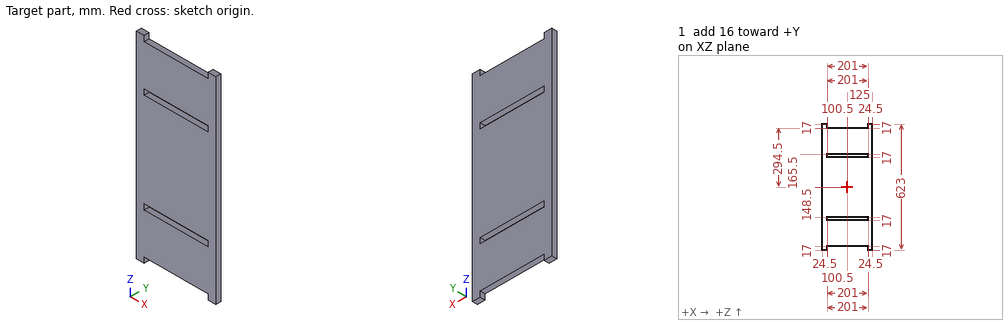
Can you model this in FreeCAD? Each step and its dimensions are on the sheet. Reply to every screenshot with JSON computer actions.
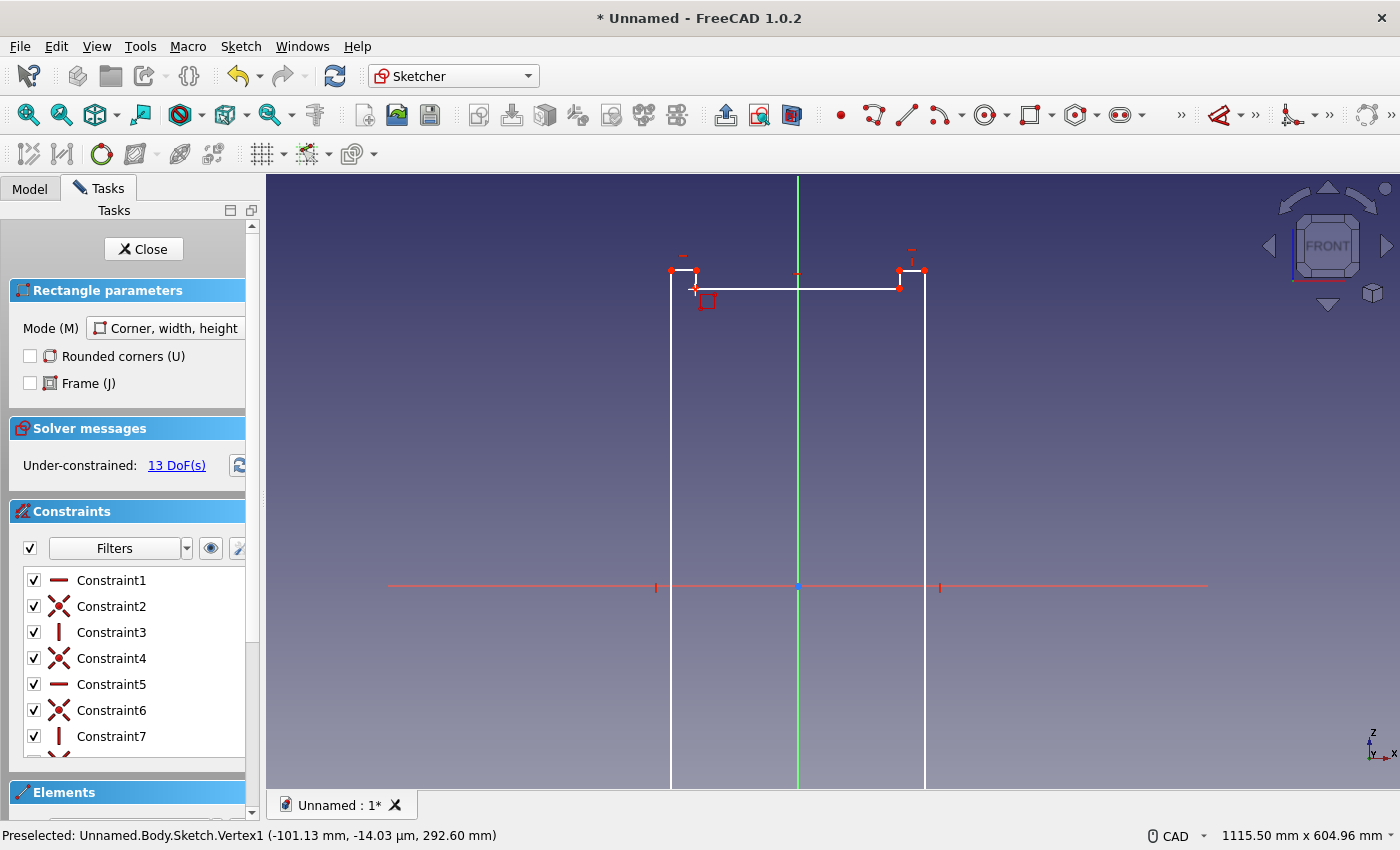
{"action": "left_click", "coordinate": [696, 418]}
{"action": "mouse_move", "coordinate": [900, 435]}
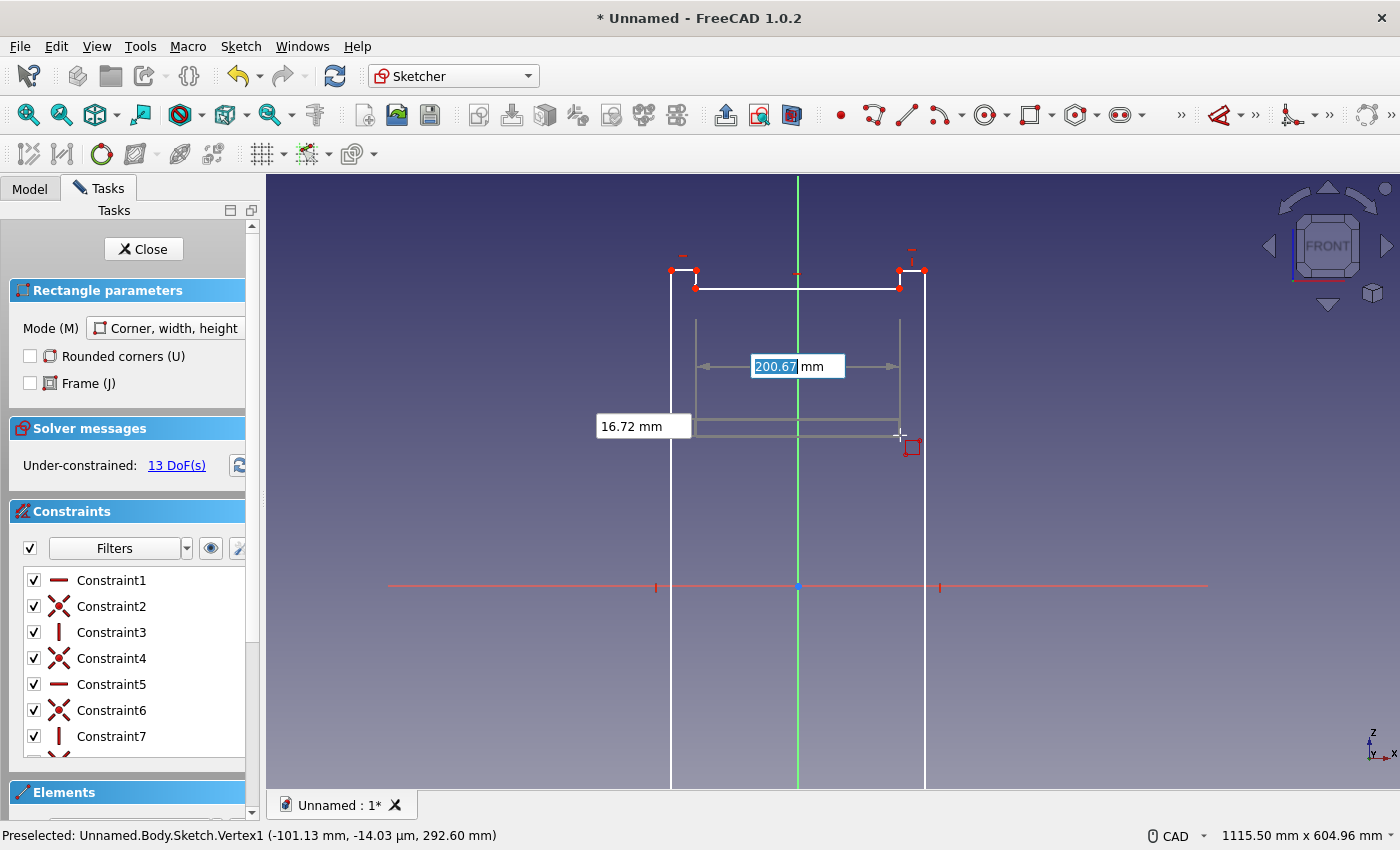
{"action": "type", "text": "201"}
{"action": "key", "text": "Tab"}
{"action": "type", "text": "17"}
{"action": "key", "text": "Return"}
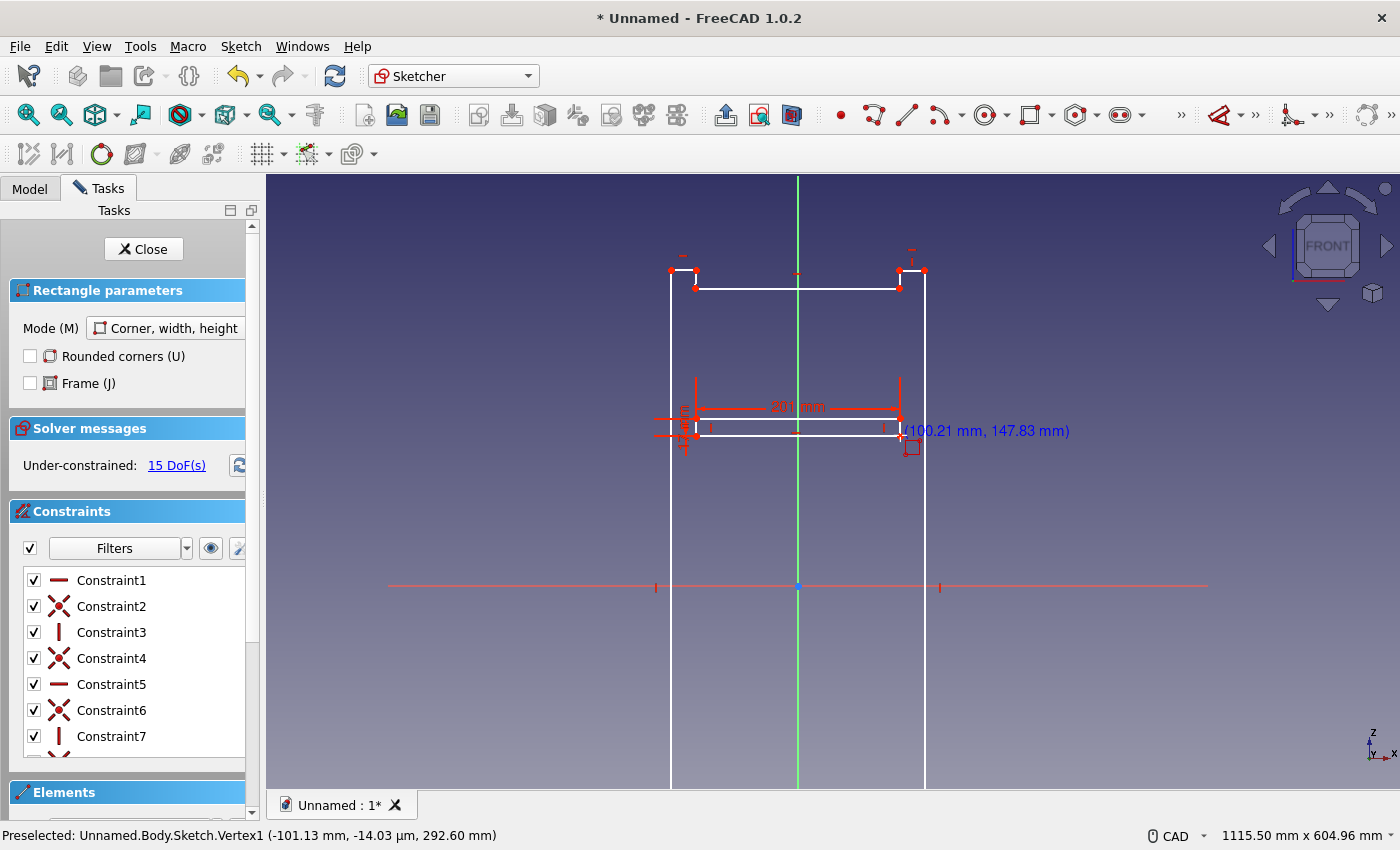
{"action": "left_click", "coordinate": [696, 737]}
{"action": "mouse_move", "coordinate": [900, 755]}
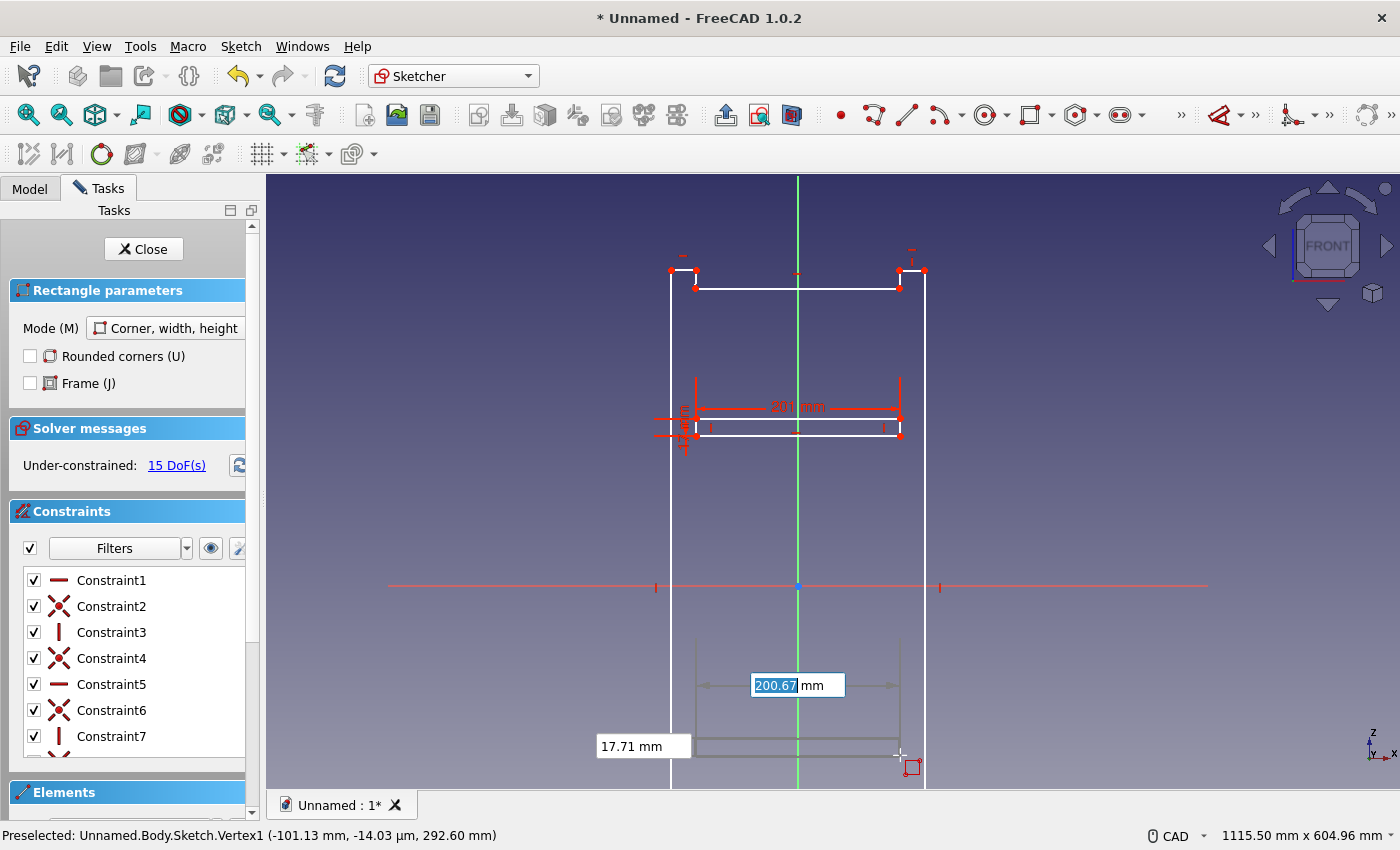
{"action": "type", "text": "201"}
{"action": "key", "text": "Tab"}
{"action": "type", "text": "17"}
{"action": "key", "text": "Return"}
{"action": "key", "text": "Escape"}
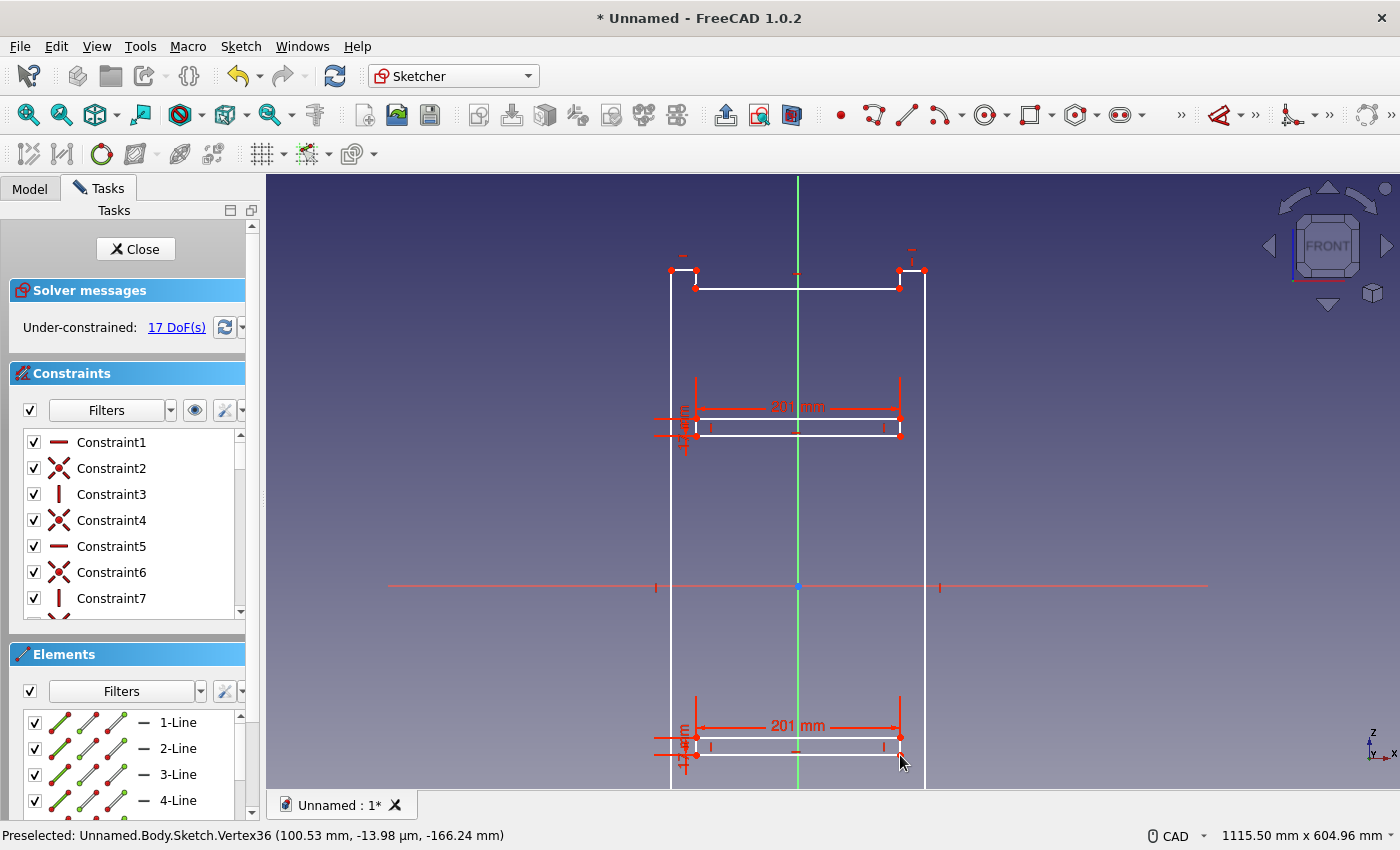
{"action": "scroll", "coordinate": [696, 280], "scroll_direction": "up", "scroll_amount": 3}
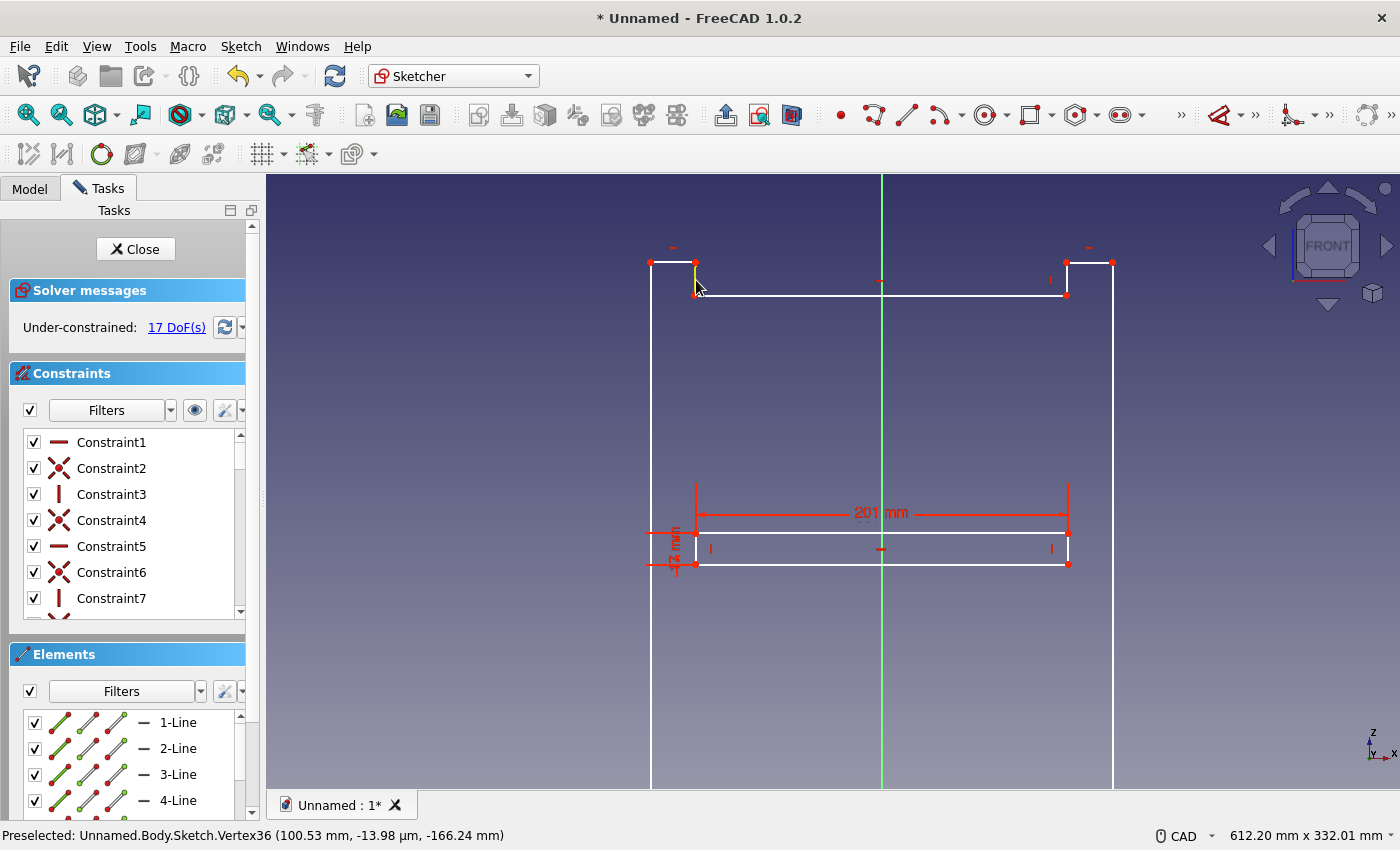
{"action": "left_click", "coordinate": [695, 279]}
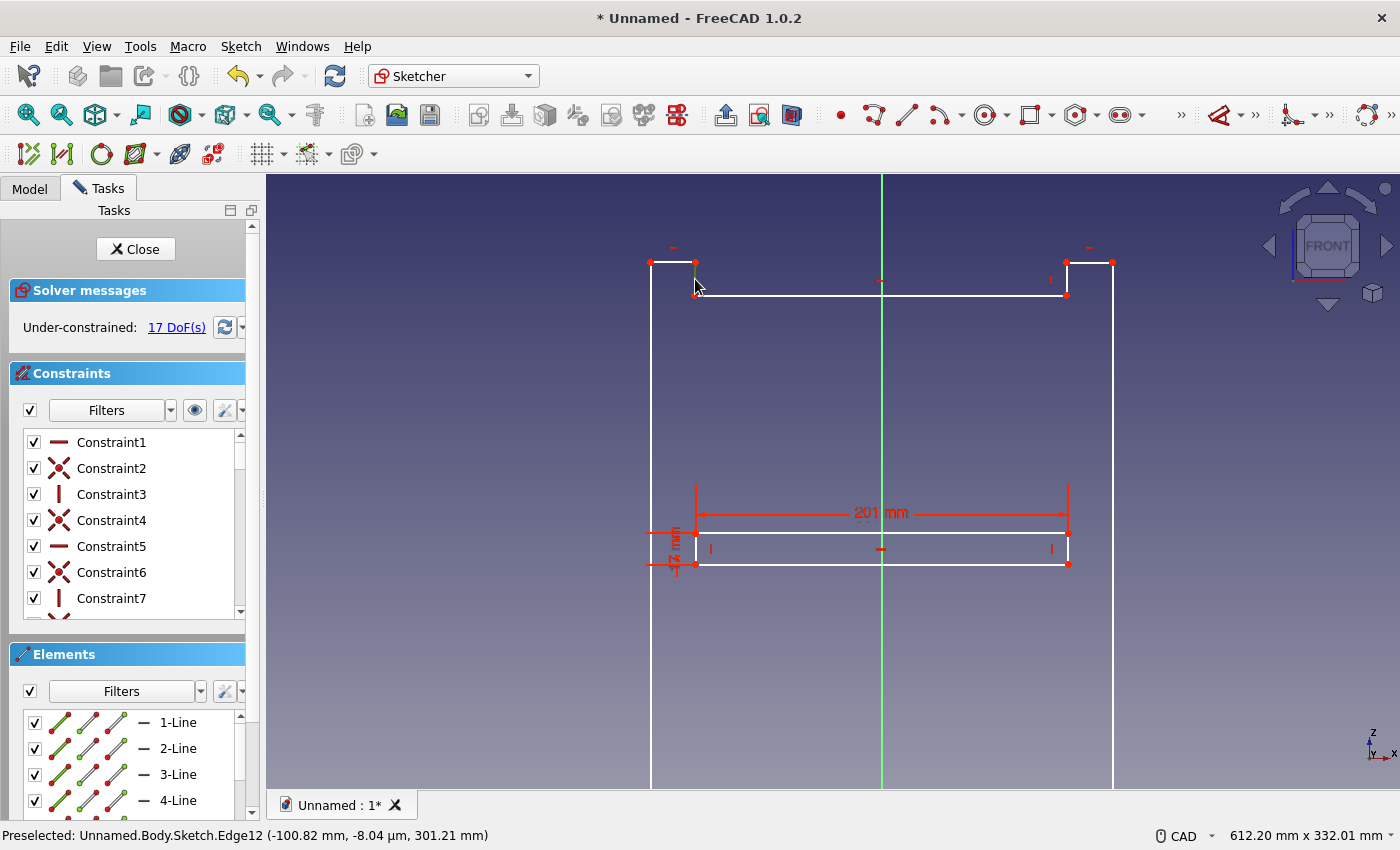
{"action": "key", "text": "v"}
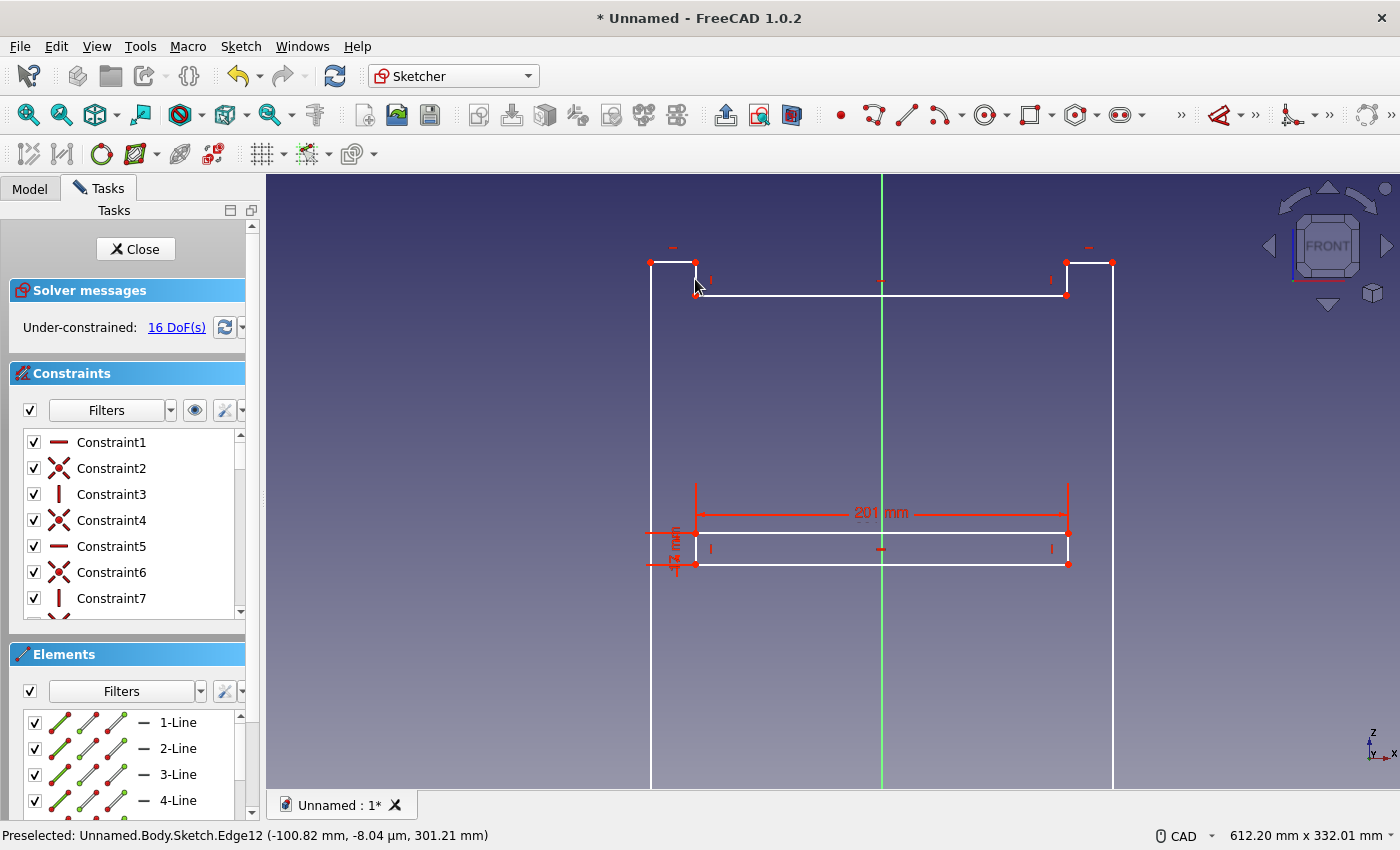
{"action": "left_click", "coordinate": [1218, 116]}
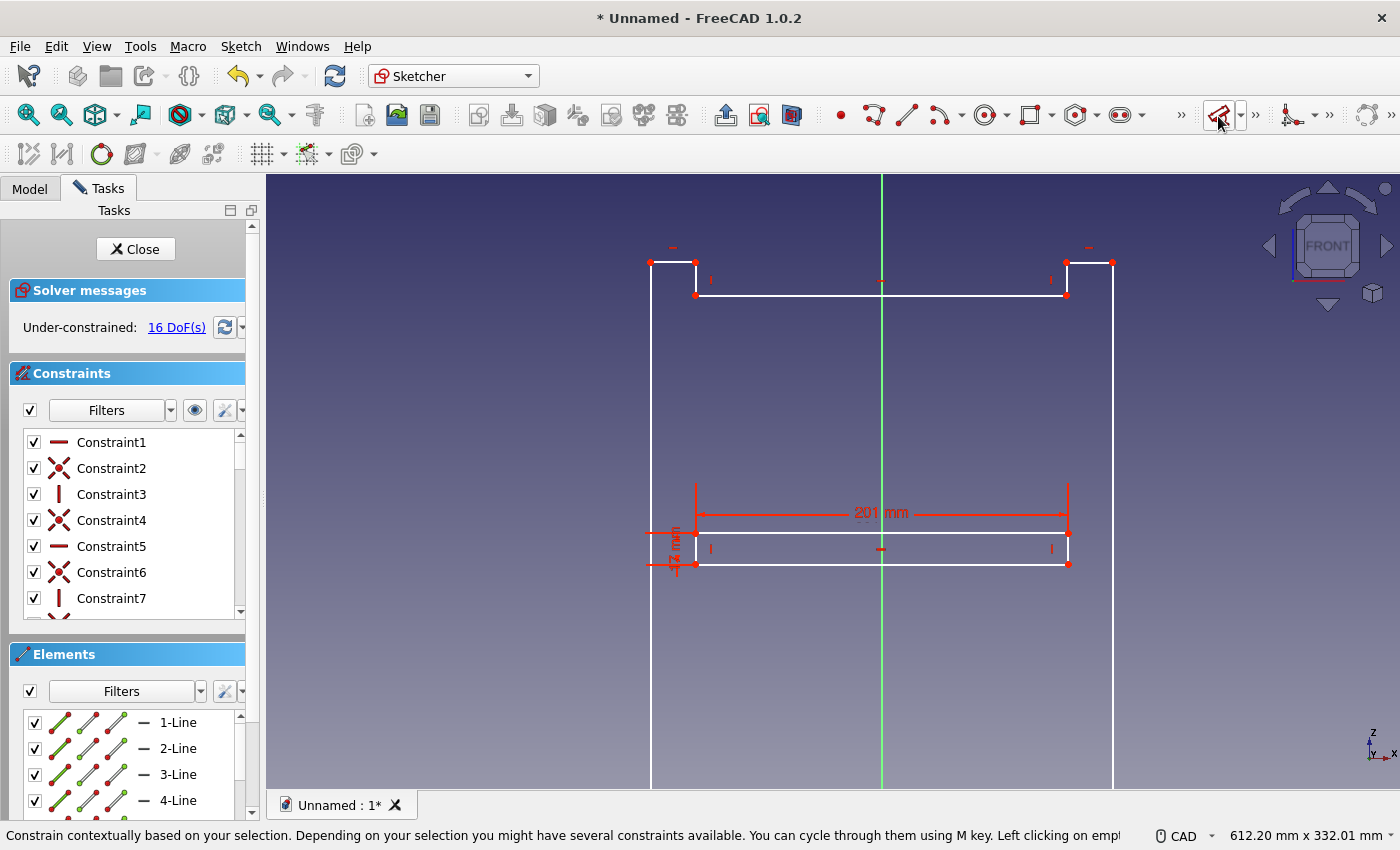
{"action": "scroll", "coordinate": [1067, 286], "scroll_direction": "up", "scroll_amount": 2}